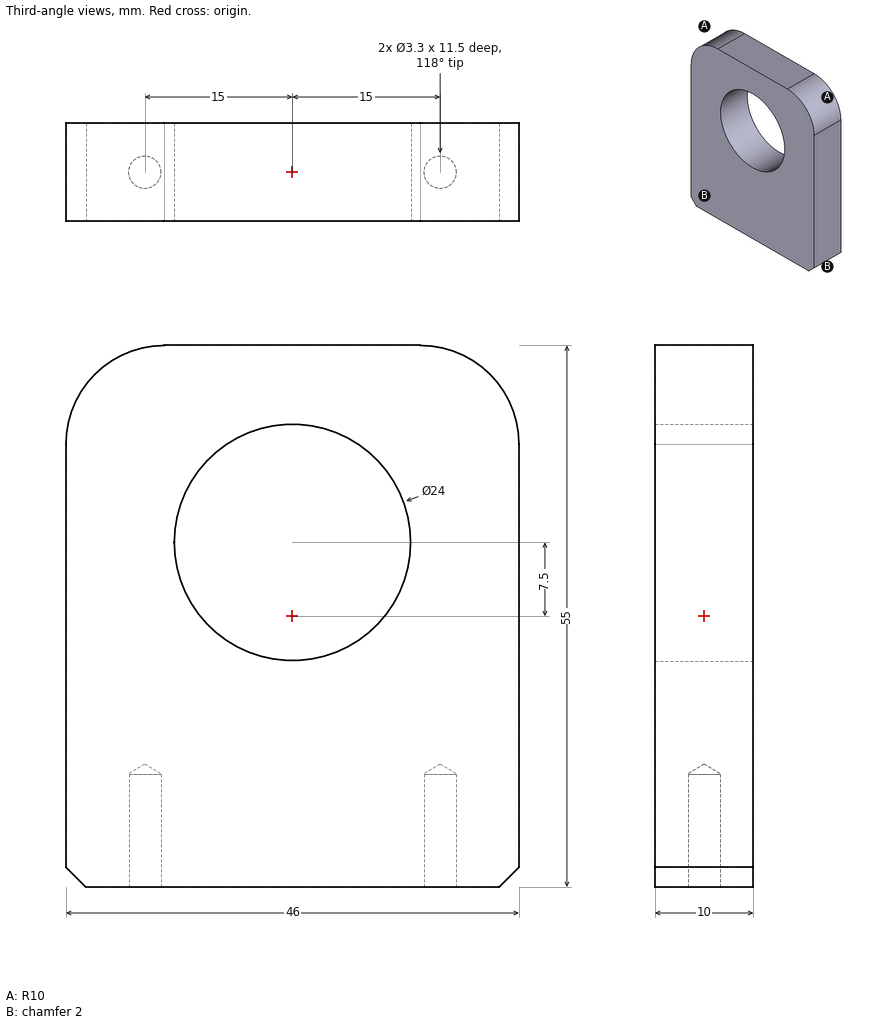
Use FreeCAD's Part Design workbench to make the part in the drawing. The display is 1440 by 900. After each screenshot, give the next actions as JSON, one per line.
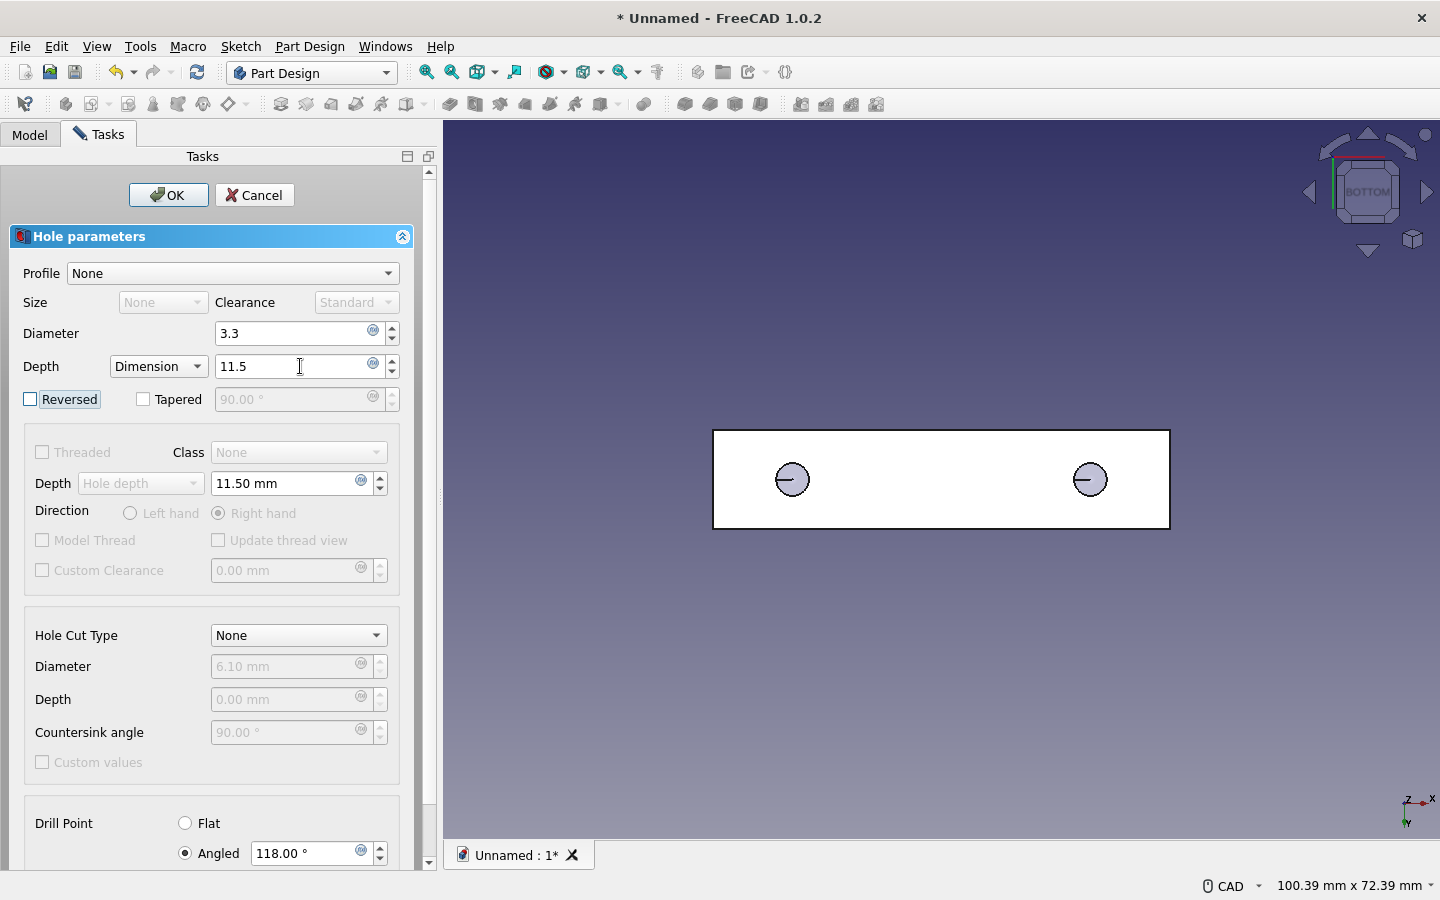
{"action": "left_click", "coordinate": [169, 195]}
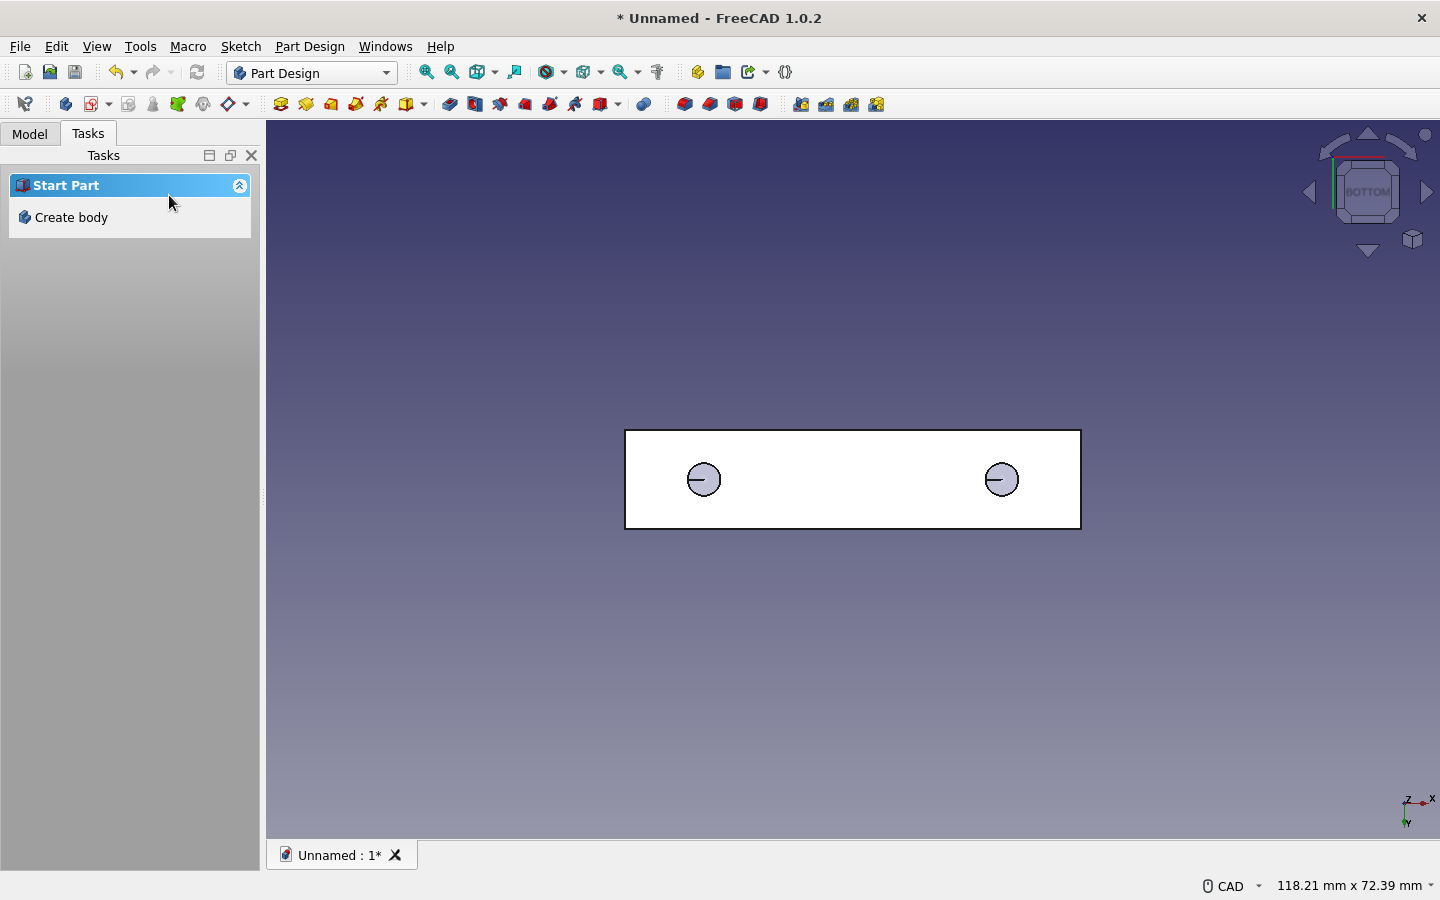
{"action": "left_click", "coordinate": [427, 72]}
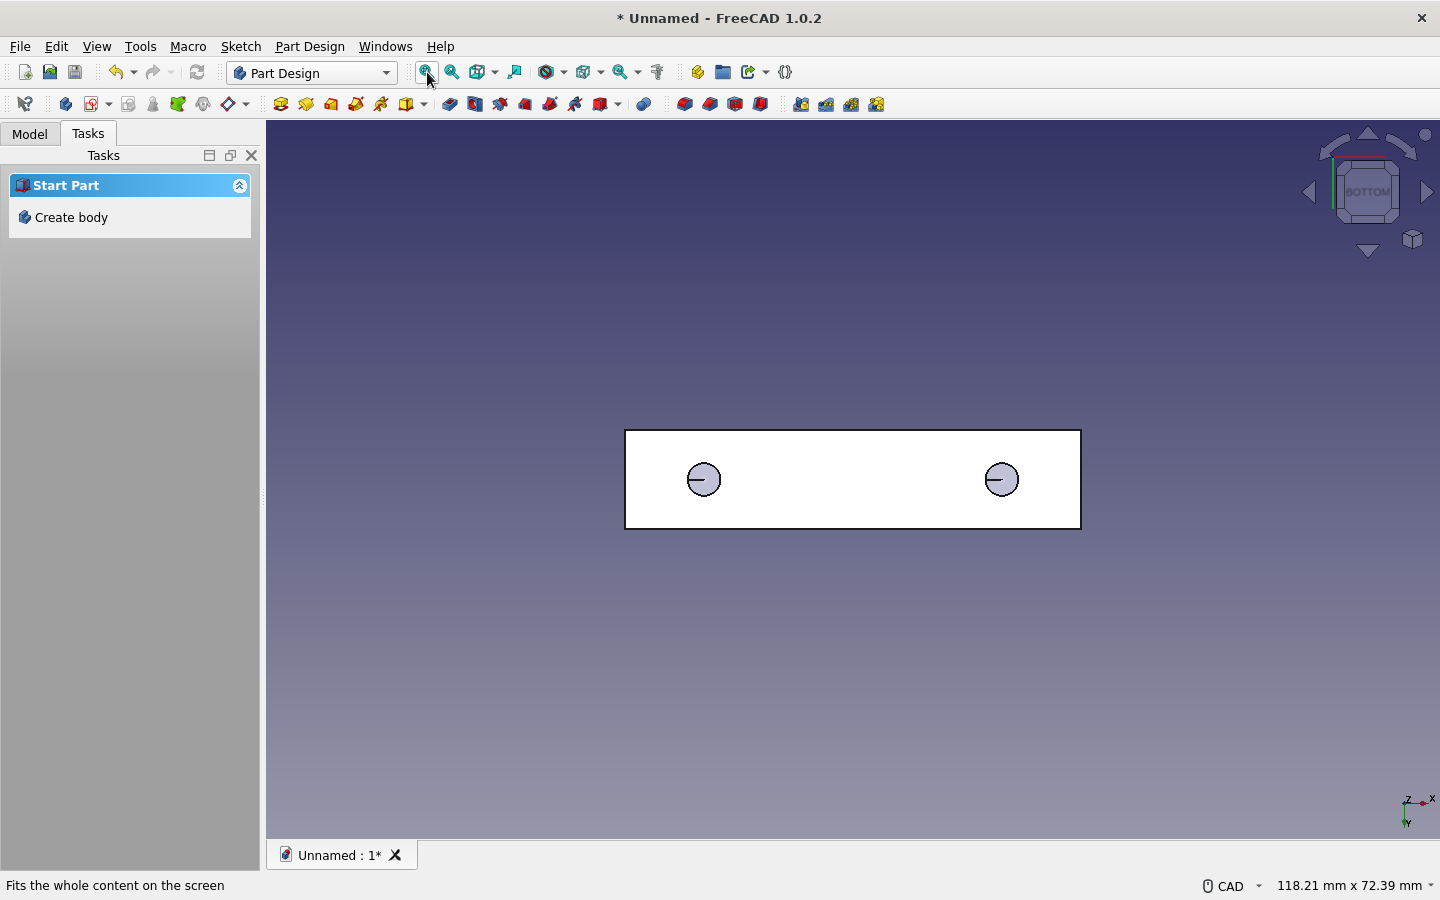
{"action": "left_click", "coordinate": [625, 478]}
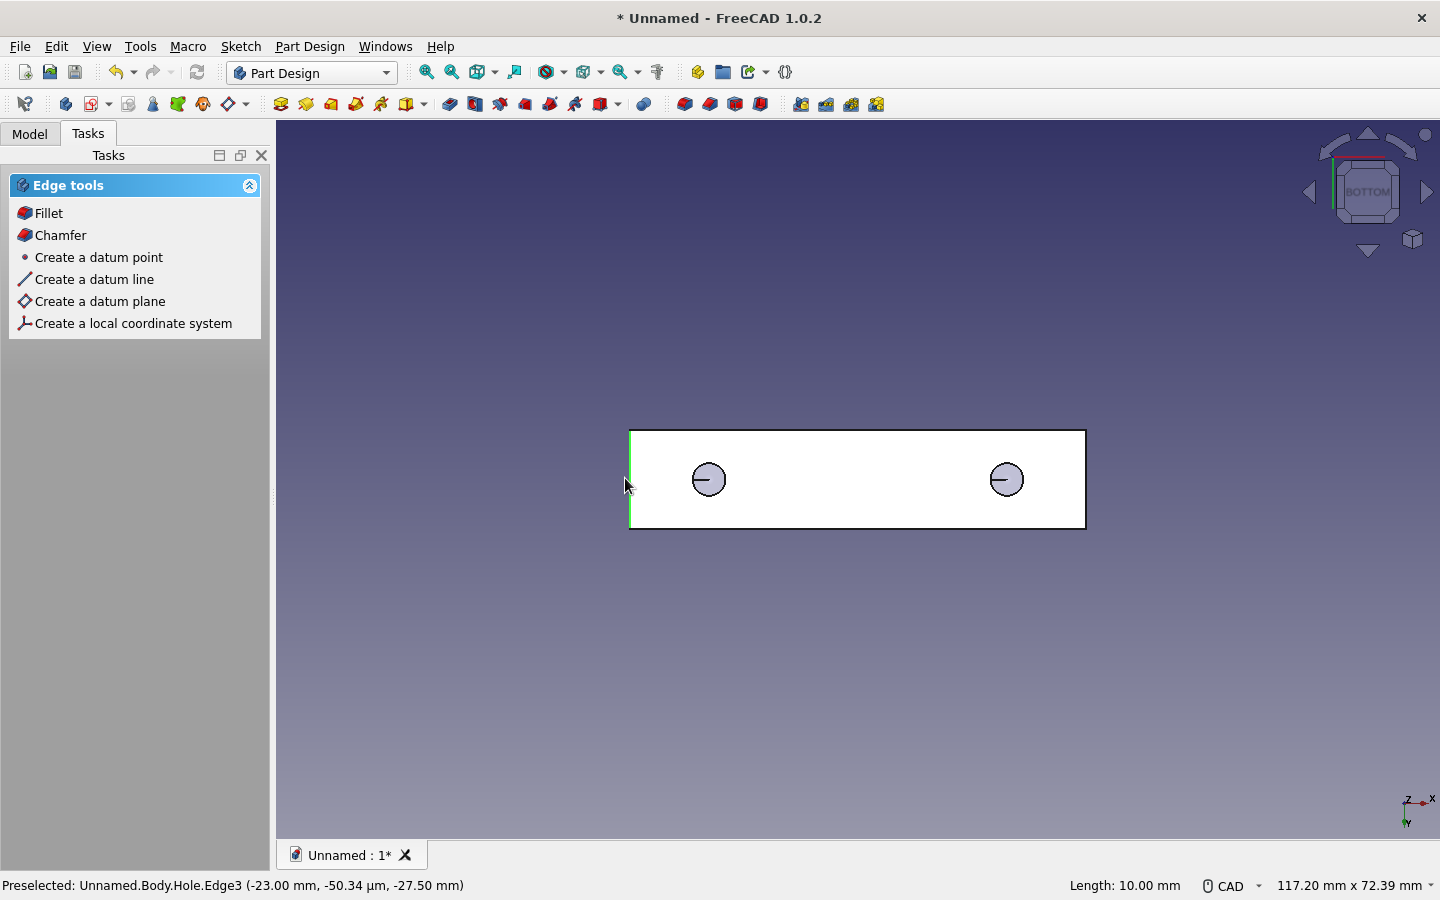
{"action": "left_click", "coordinate": [1086, 478], "text": "ctrl"}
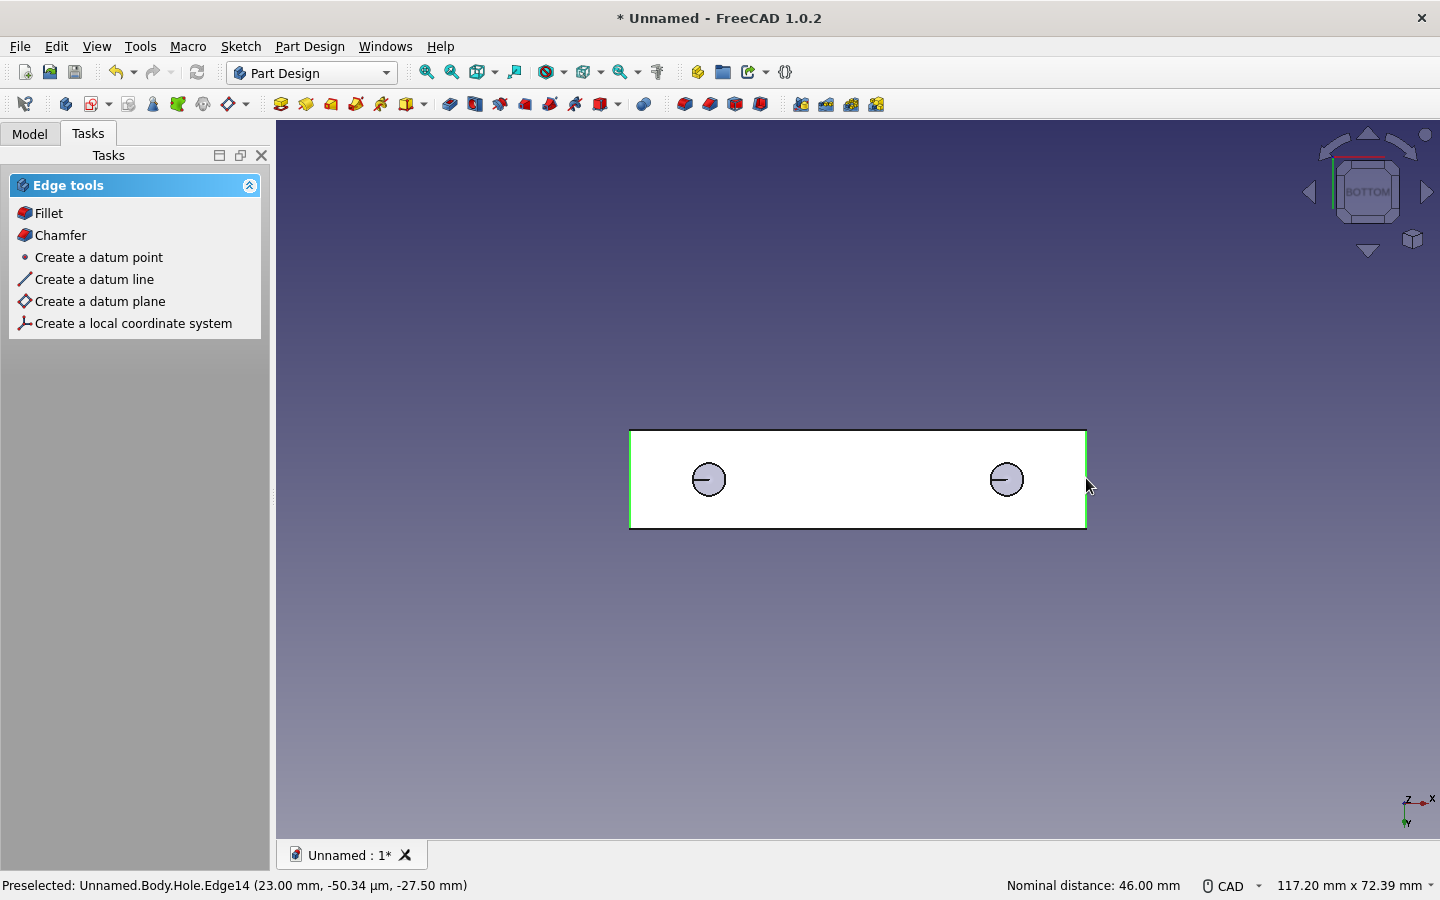
{"action": "left_click", "coordinate": [710, 104]}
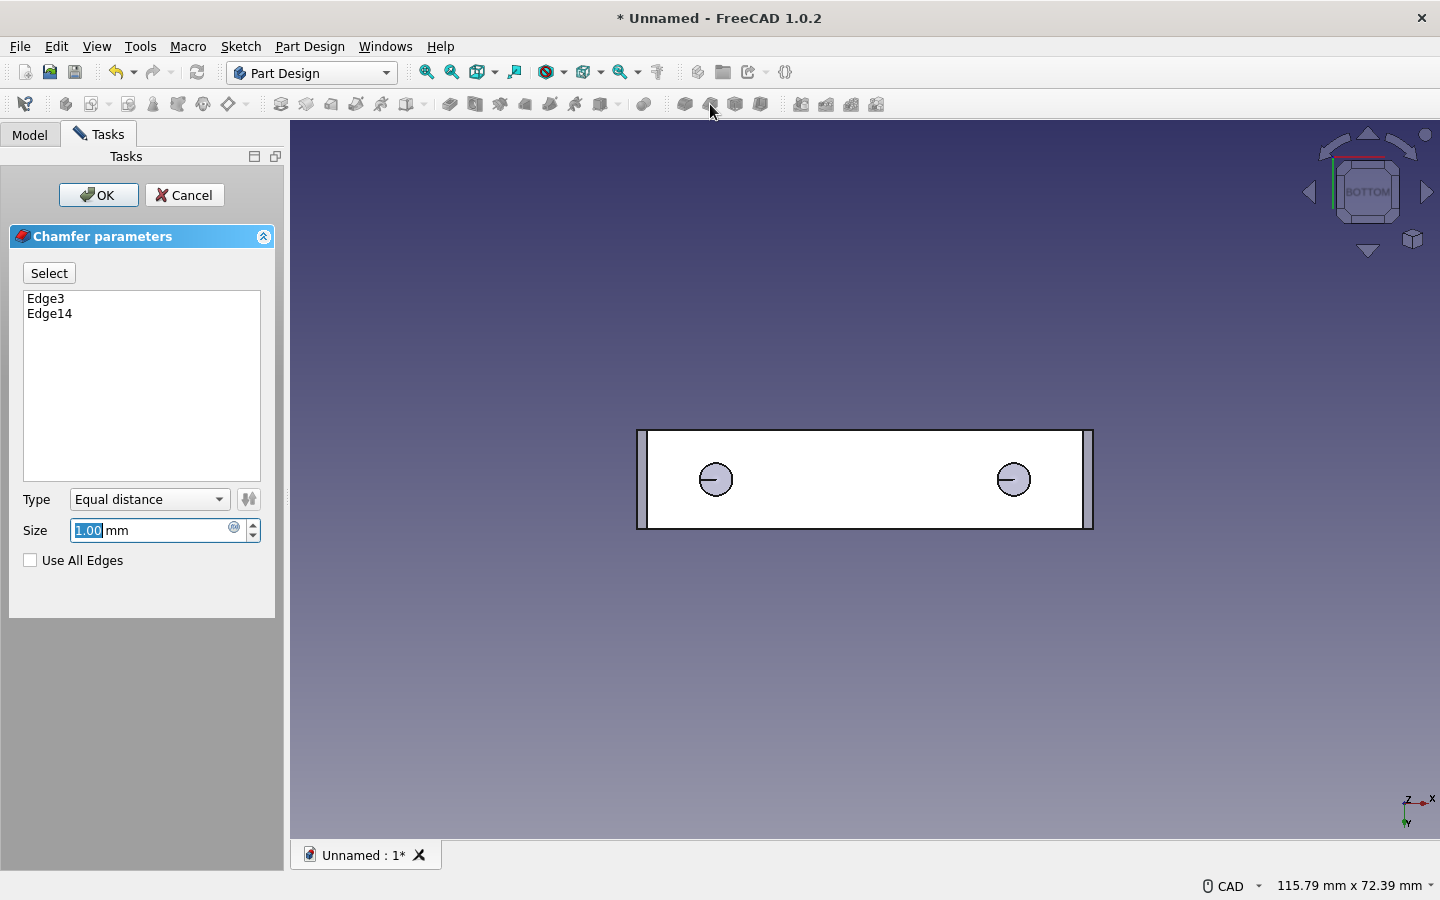
{"action": "type", "text": "2"}
{"action": "key", "text": "Tab"}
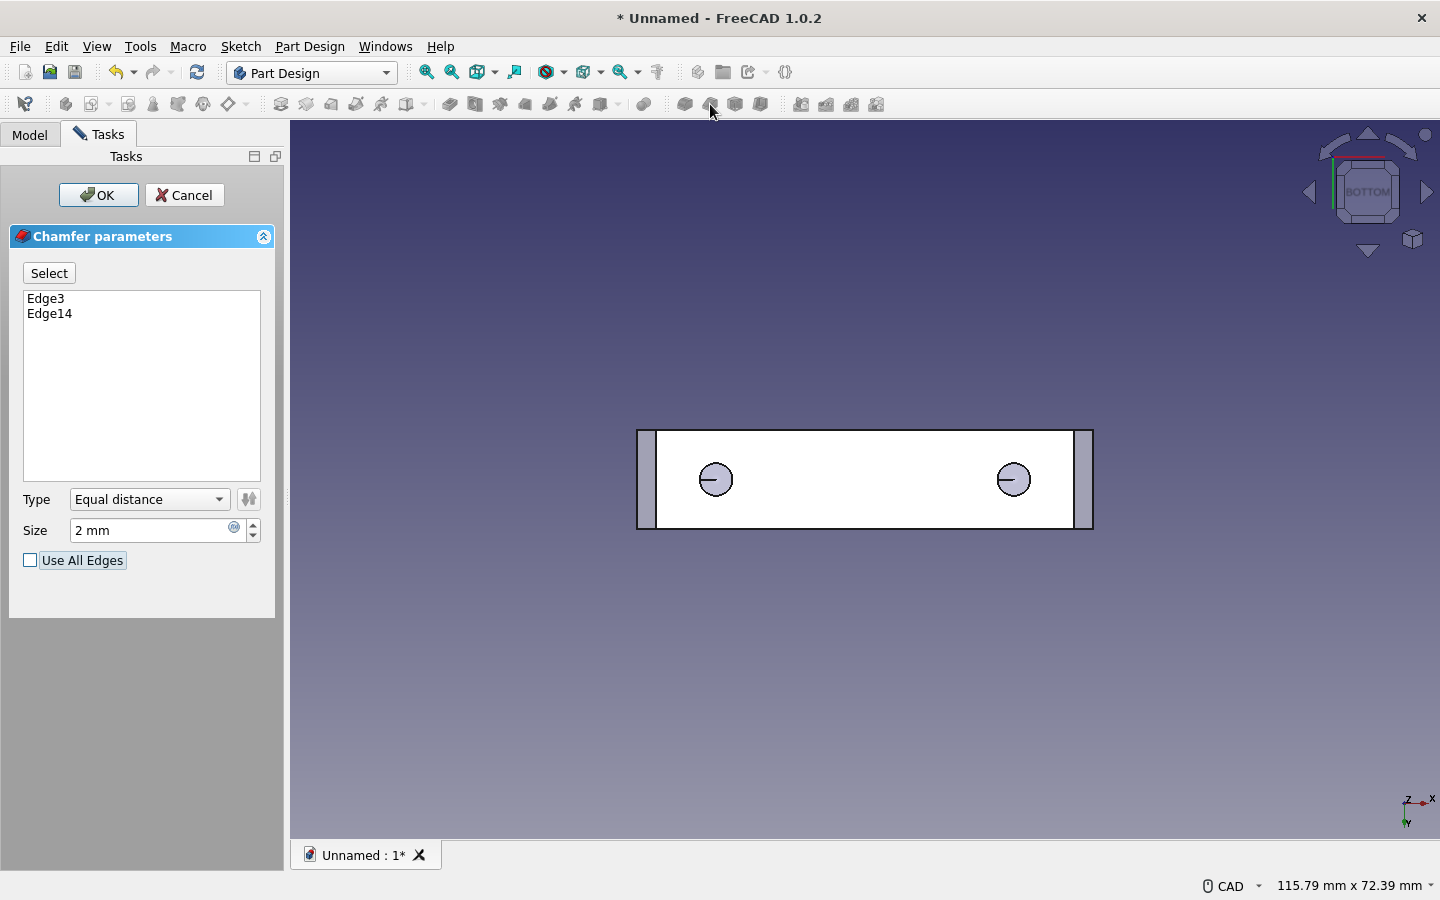
{"action": "left_click", "coordinate": [99, 195]}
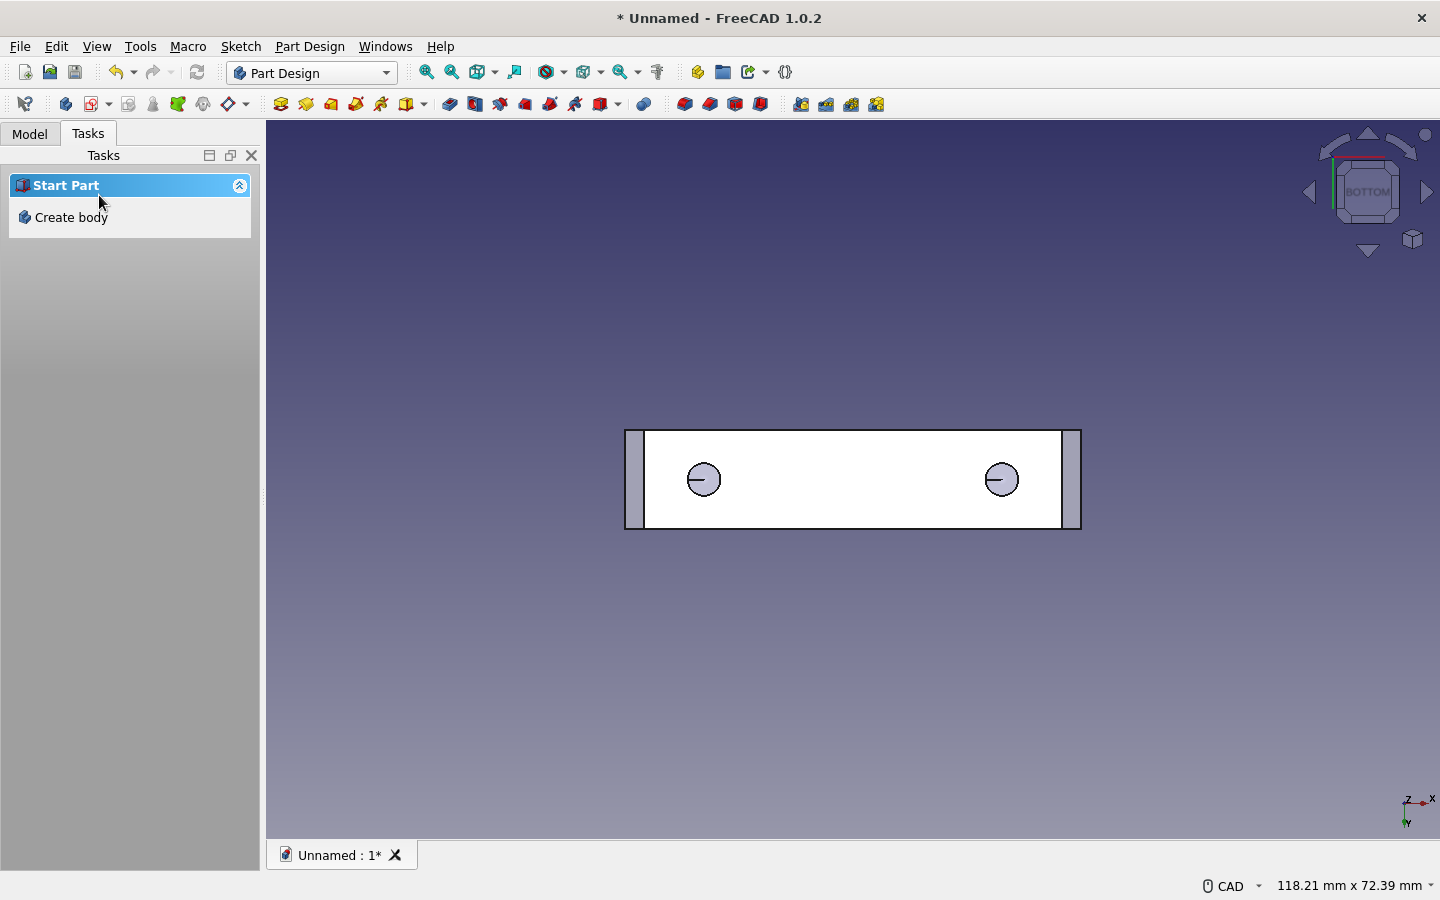
{"action": "key", "text": "0"}